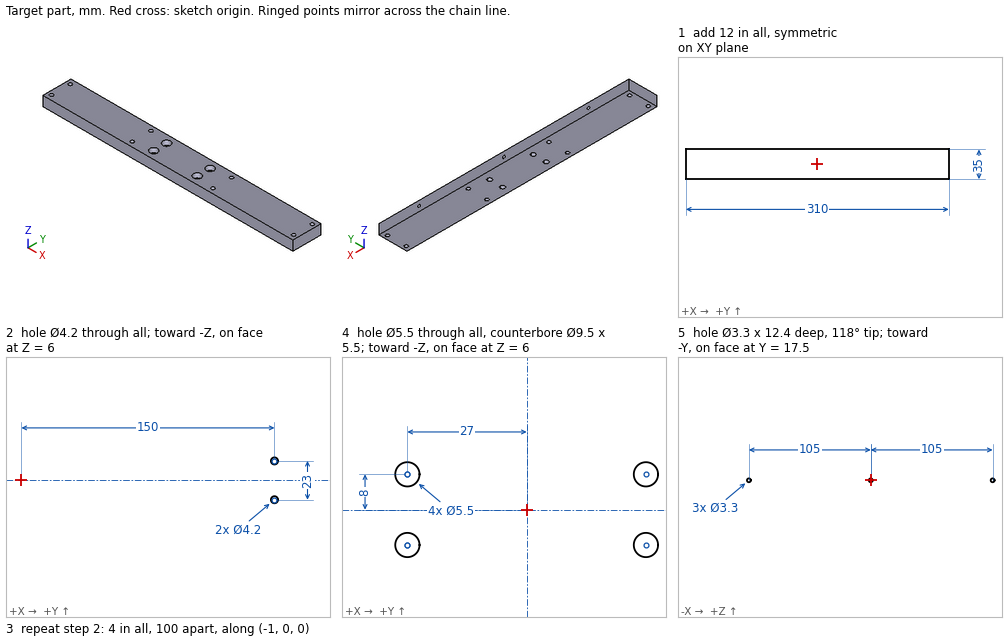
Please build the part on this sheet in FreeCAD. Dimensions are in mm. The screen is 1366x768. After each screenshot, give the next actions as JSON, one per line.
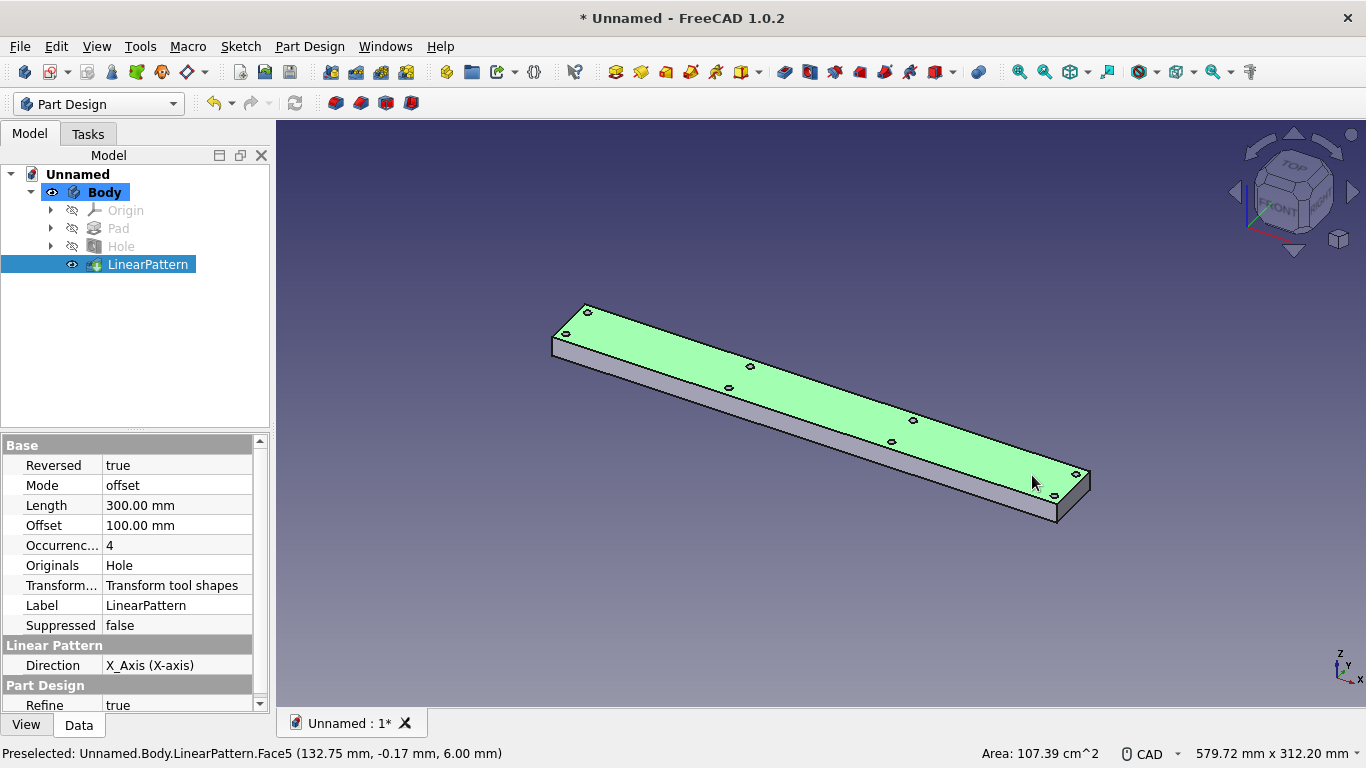
{"action": "left_click", "coordinate": [50, 72]}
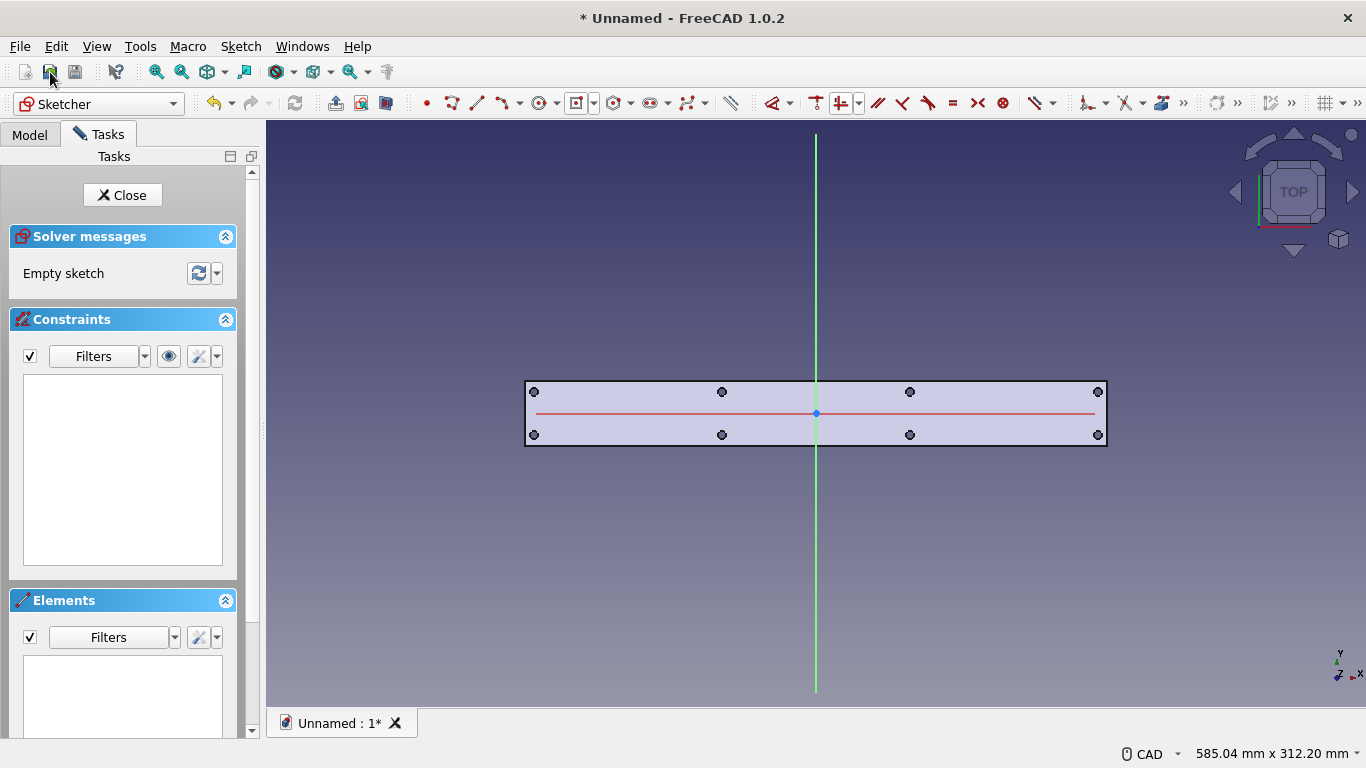
{"action": "scroll", "coordinate": [830, 414], "scroll_direction": "up", "scroll_amount": 9}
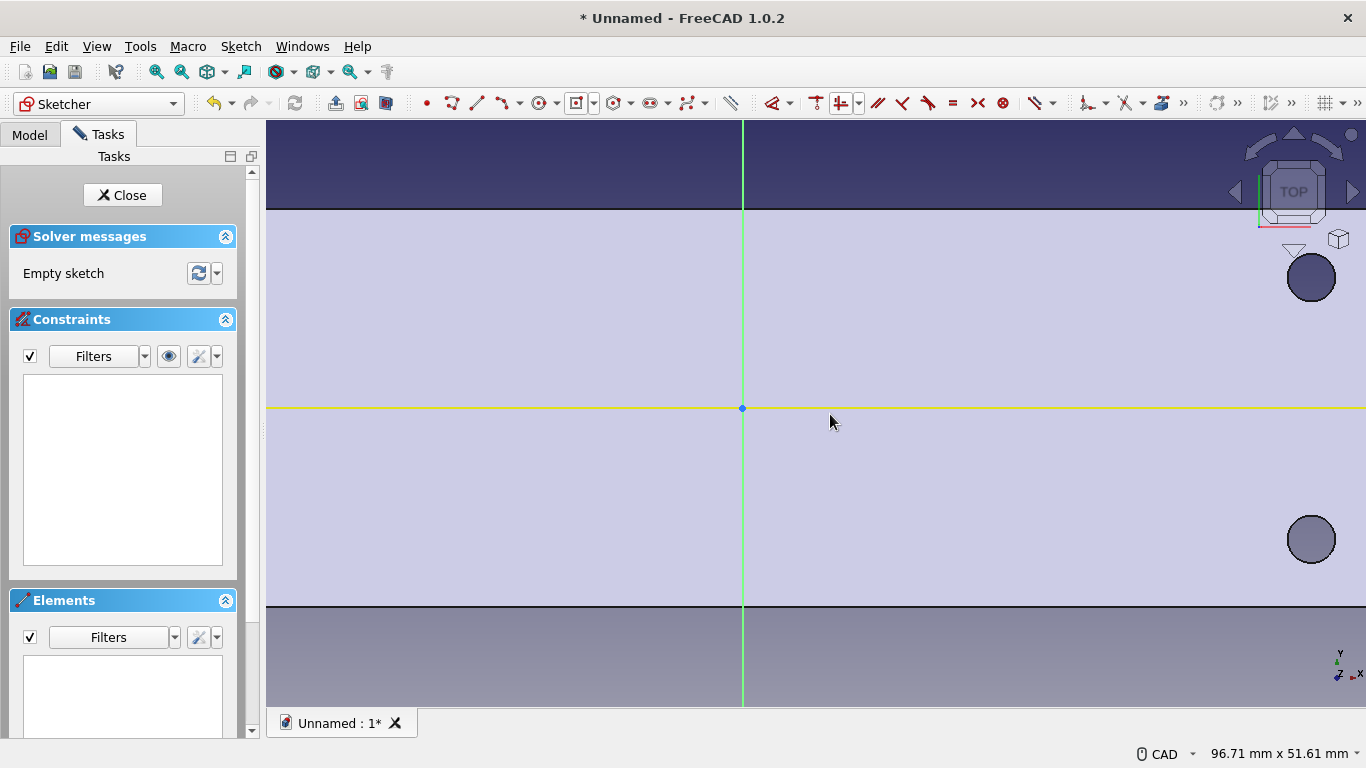
{"action": "left_click", "coordinate": [538, 104]}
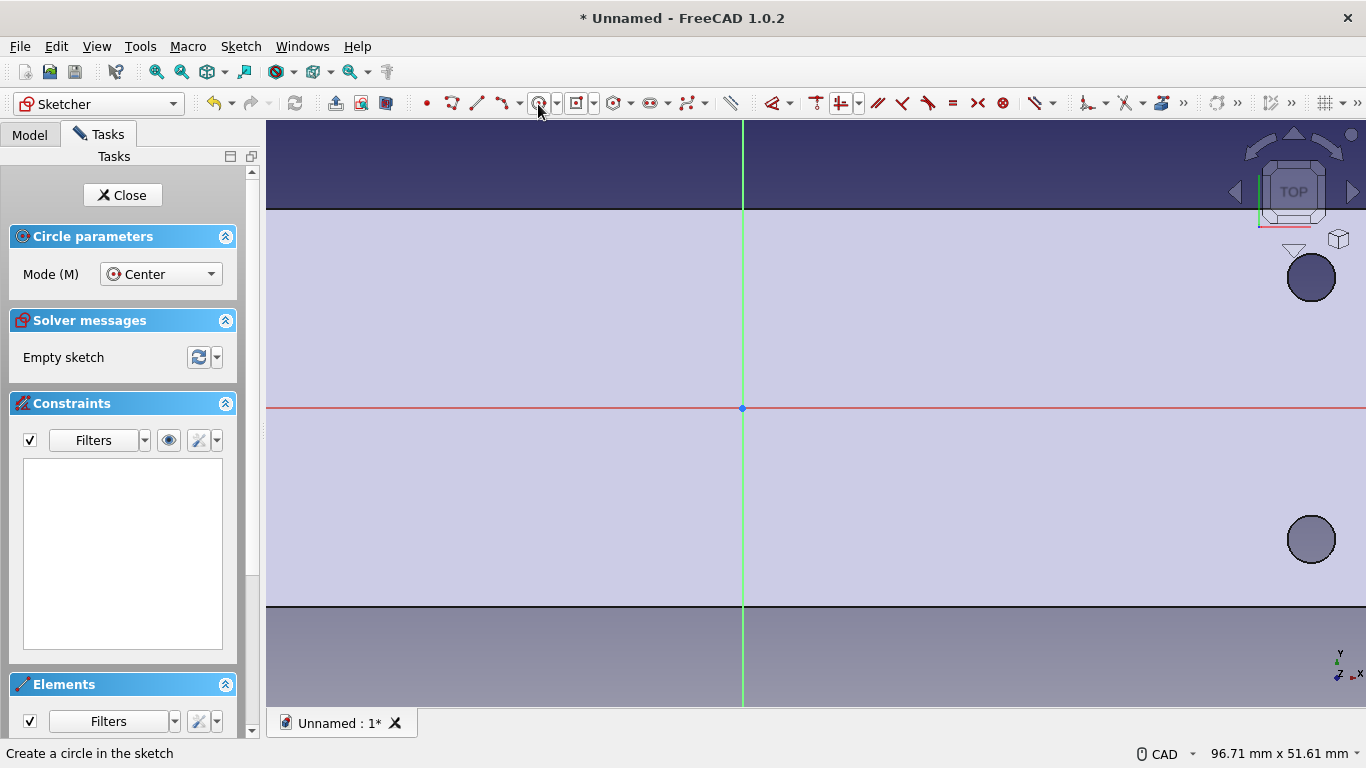
{"action": "left_click", "coordinate": [436, 317]}
{"action": "left_click", "coordinate": [458, 295]}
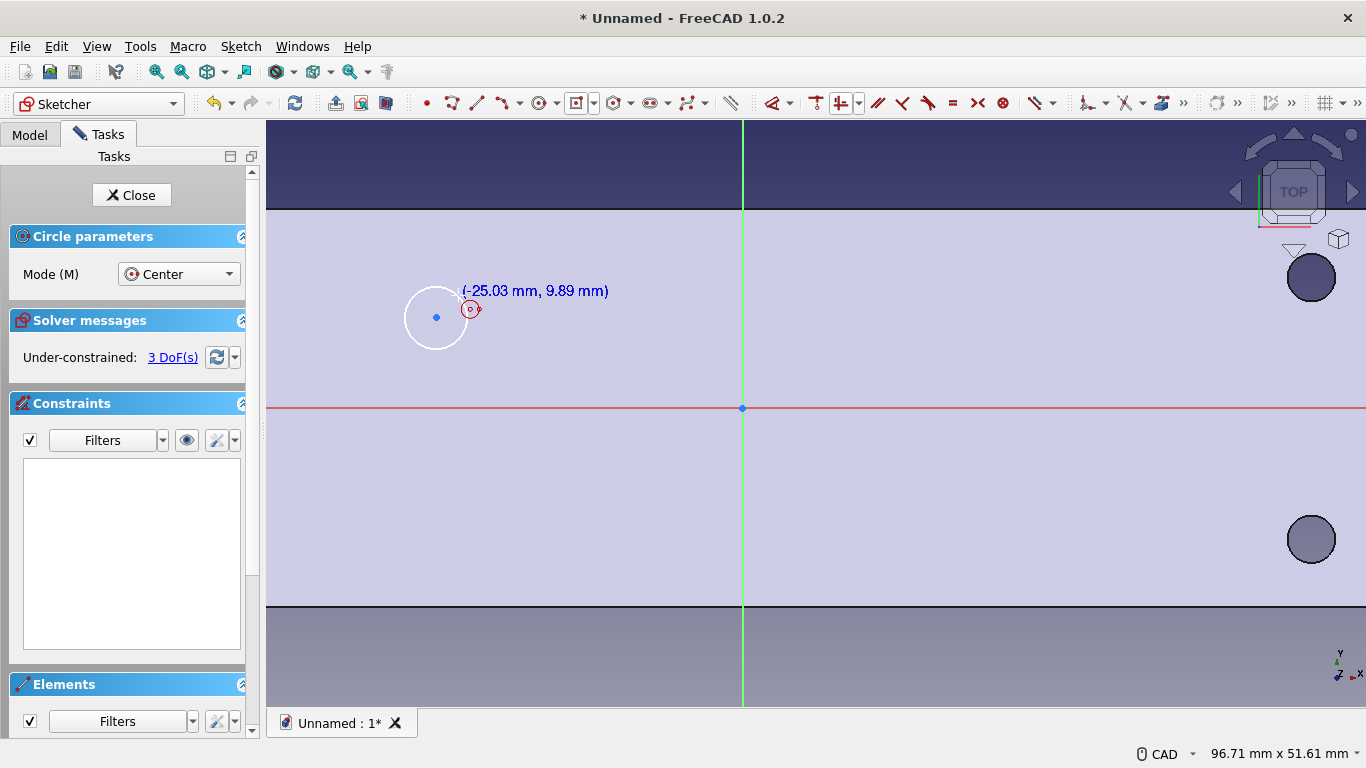
{"action": "left_click", "coordinate": [436, 499]}
{"action": "left_click", "coordinate": [458, 477]}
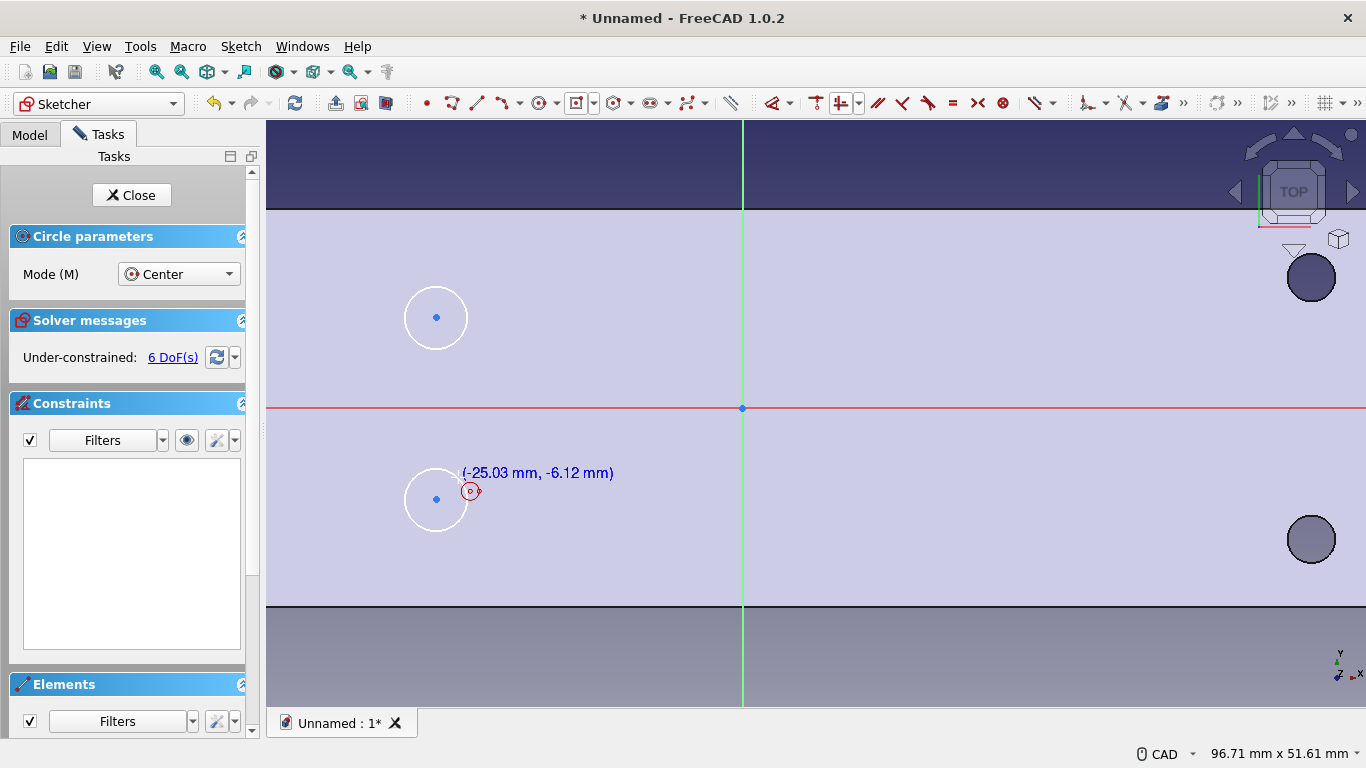
{"action": "left_click", "coordinate": [1050, 317]}
{"action": "left_click", "coordinate": [1072, 295]}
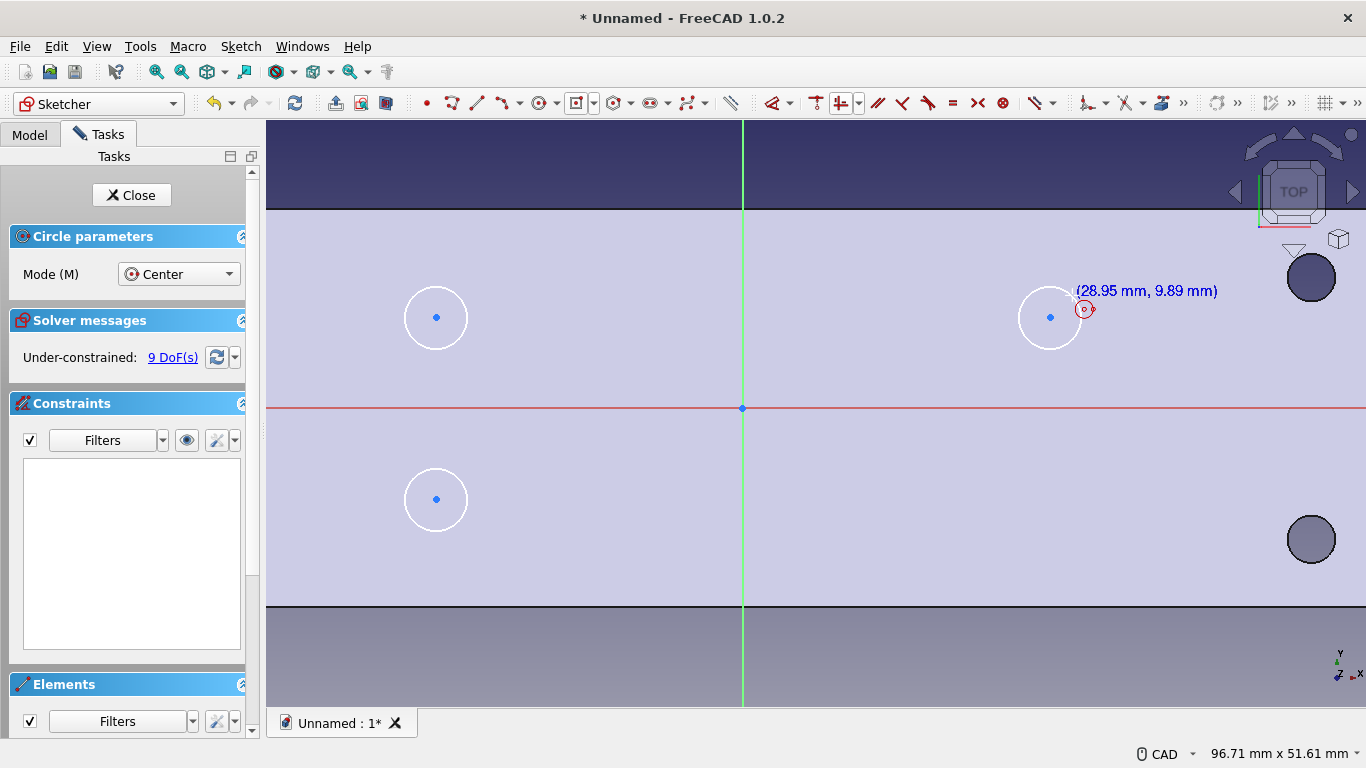
{"action": "left_click", "coordinate": [1050, 499]}
{"action": "left_click", "coordinate": [1072, 477]}
{"action": "key", "text": "Escape"}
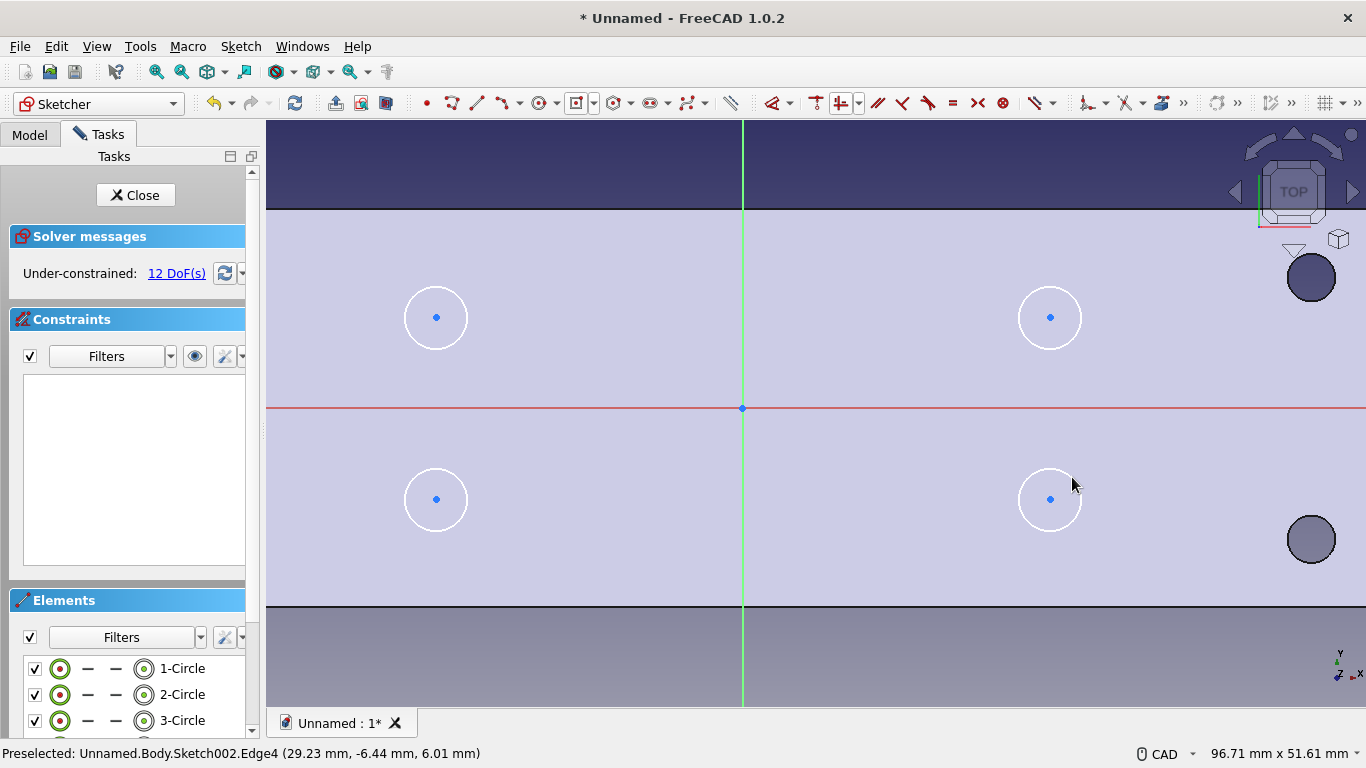
{"action": "left_click", "coordinate": [458, 296]}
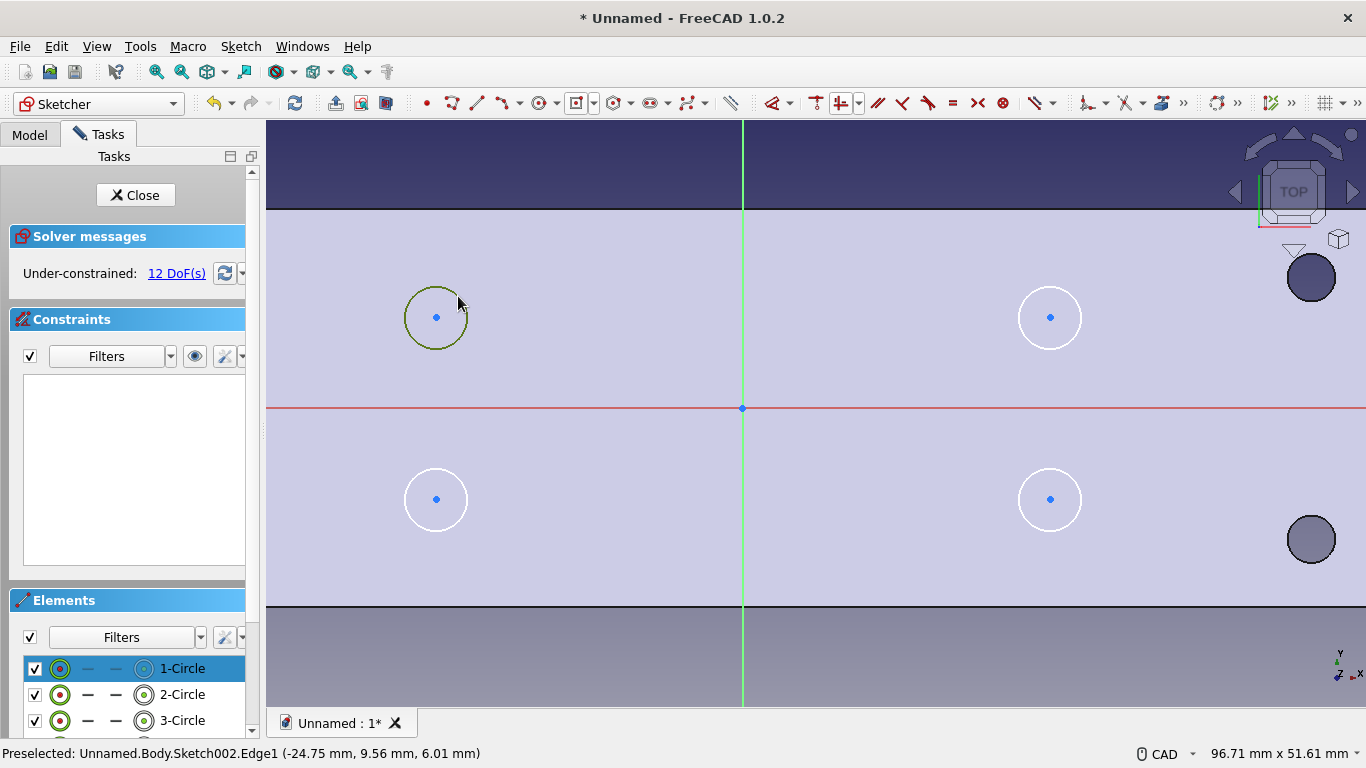
{"action": "left_click", "coordinate": [458, 478]}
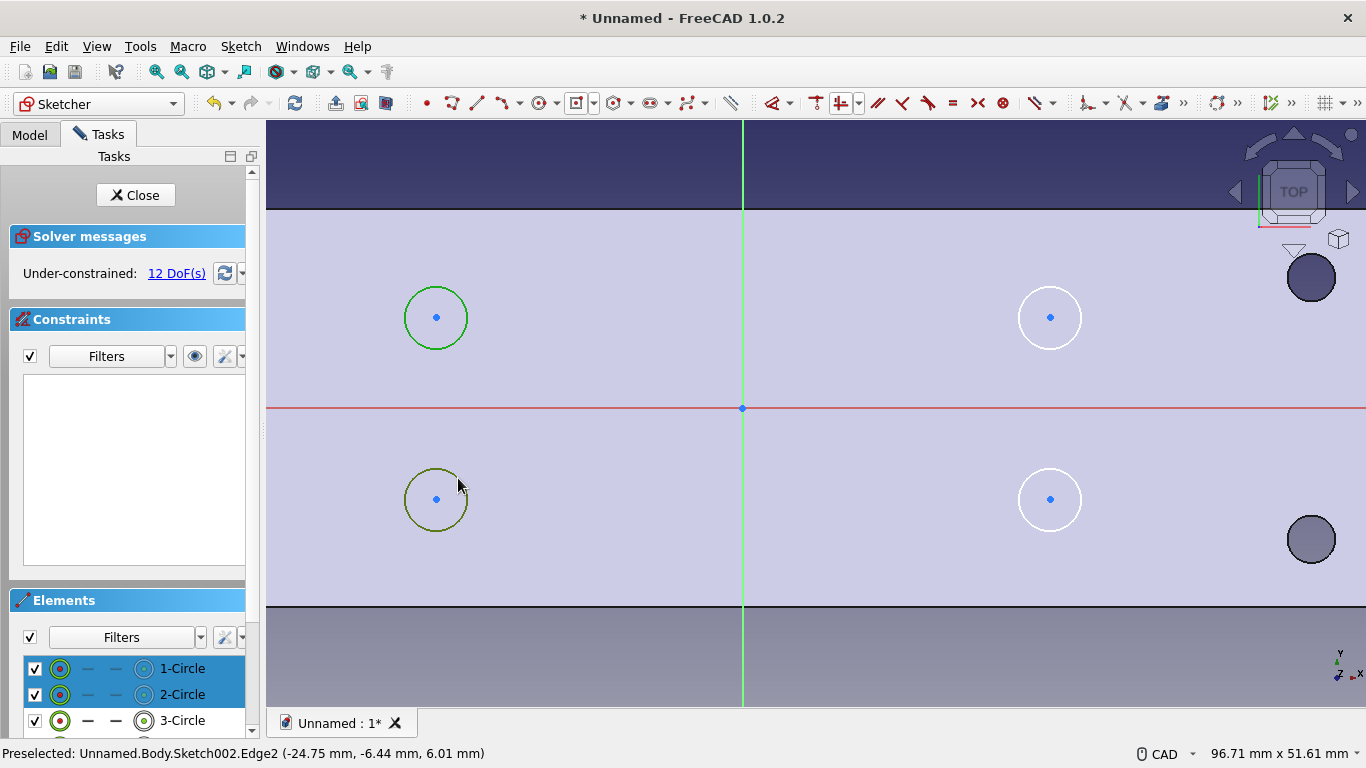
{"action": "left_click", "coordinate": [1072, 296]}